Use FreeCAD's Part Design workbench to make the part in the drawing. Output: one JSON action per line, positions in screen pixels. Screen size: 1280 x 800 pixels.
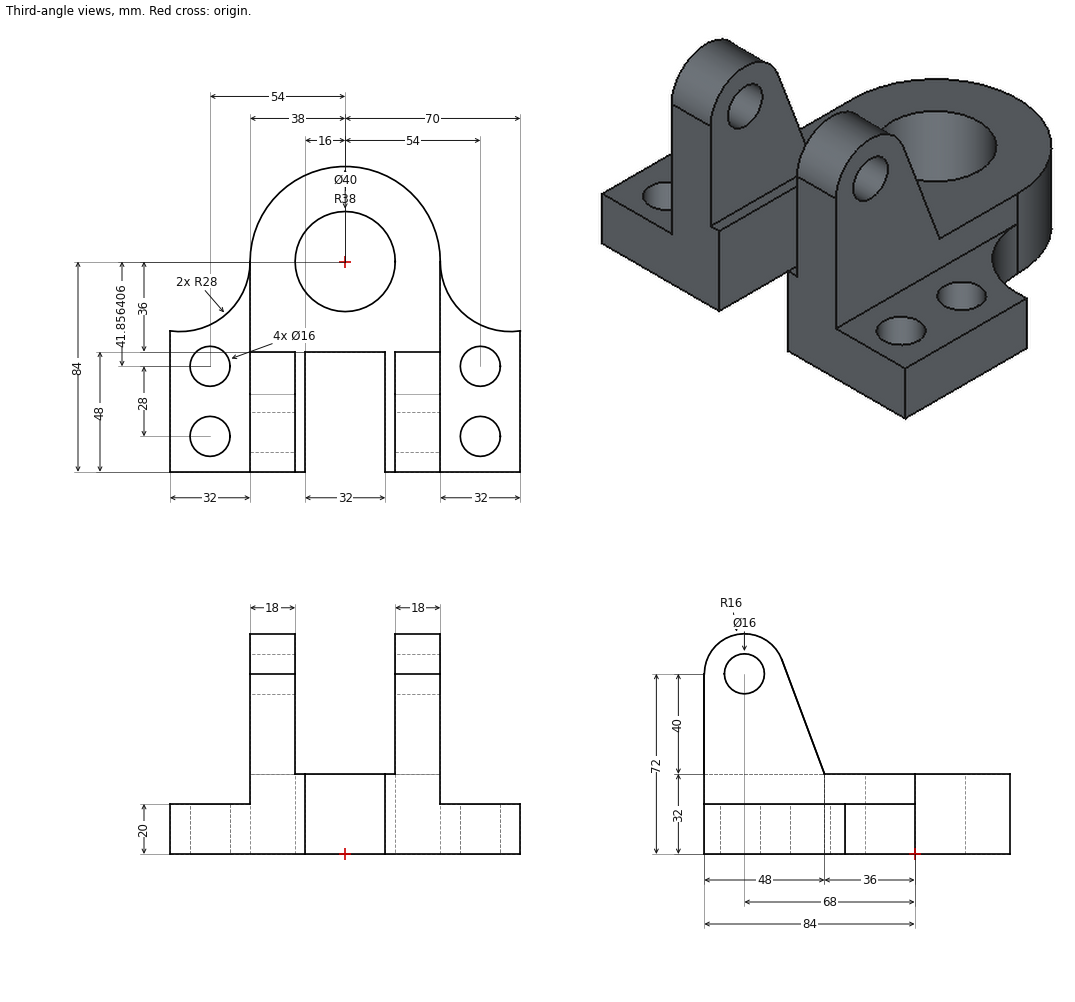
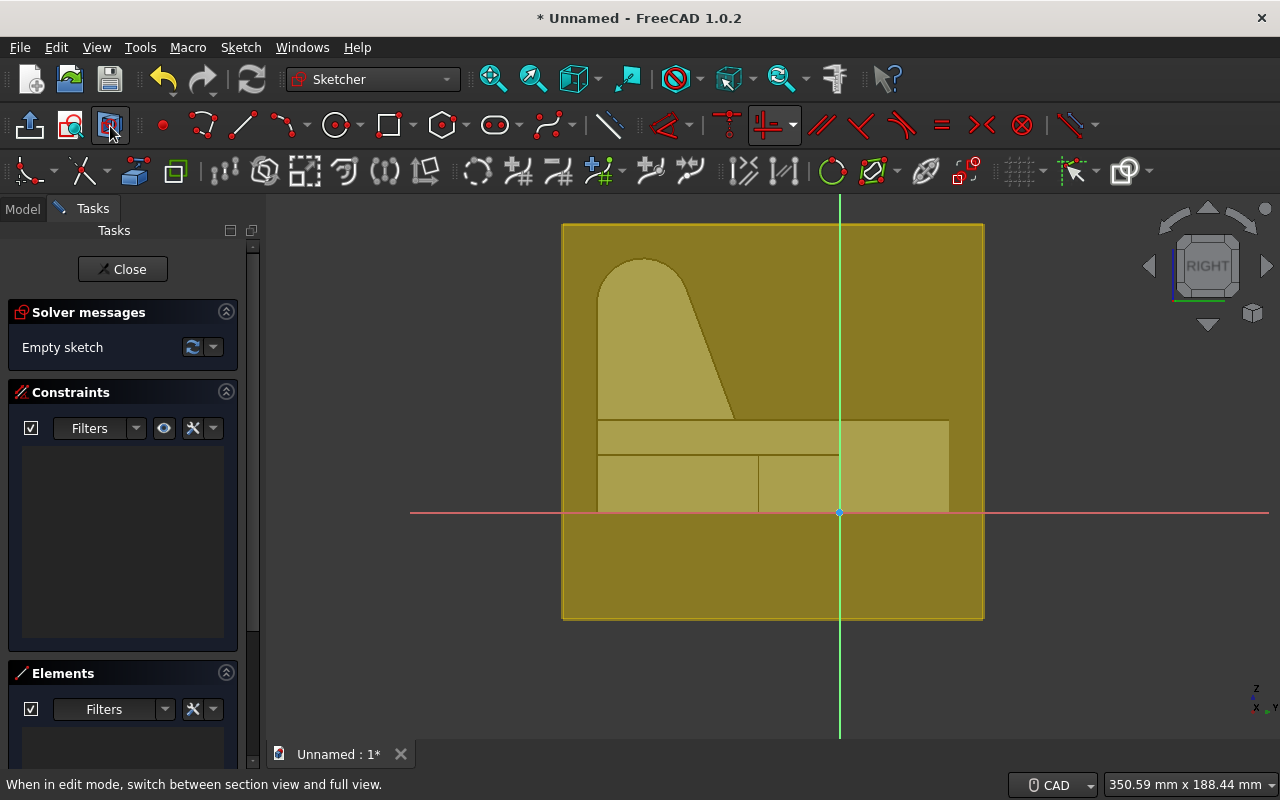
{"action": "scroll", "coordinate": [746, 222], "scroll_direction": "up", "scroll_amount": 2}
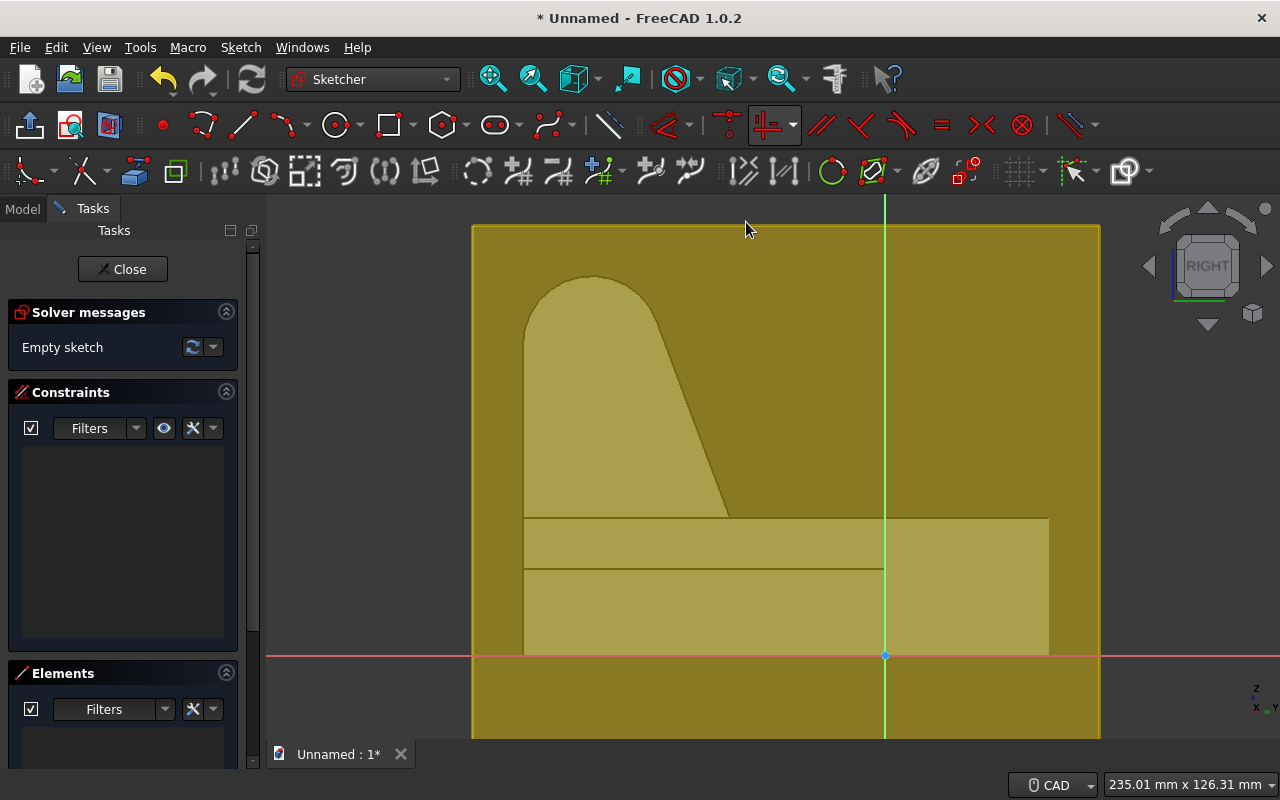
{"action": "left_click", "coordinate": [204, 126]}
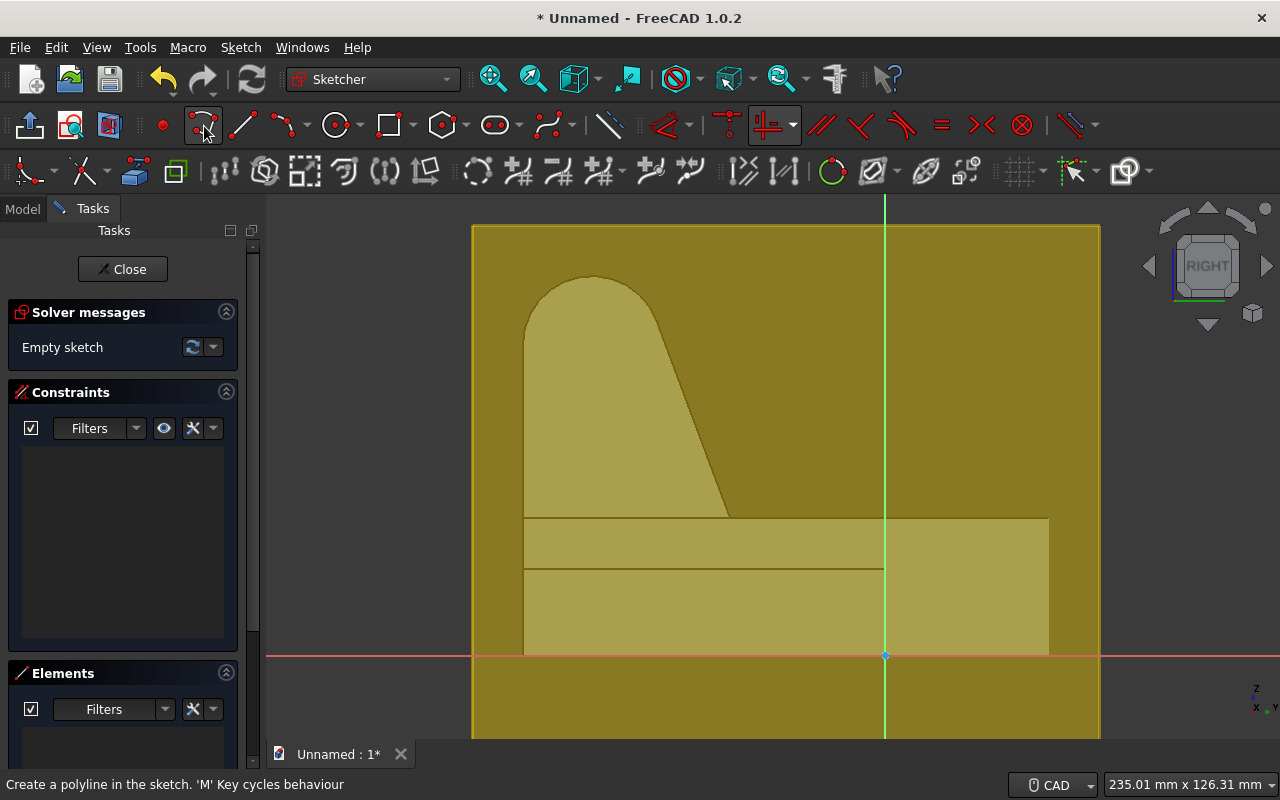
{"action": "left_click", "coordinate": [523, 345]}
{"action": "left_click", "coordinate": [523, 518]}
{"action": "left_click", "coordinate": [730, 518]}
{"action": "left_click", "coordinate": [657, 321]}
{"action": "right_click", "coordinate": [657, 321]}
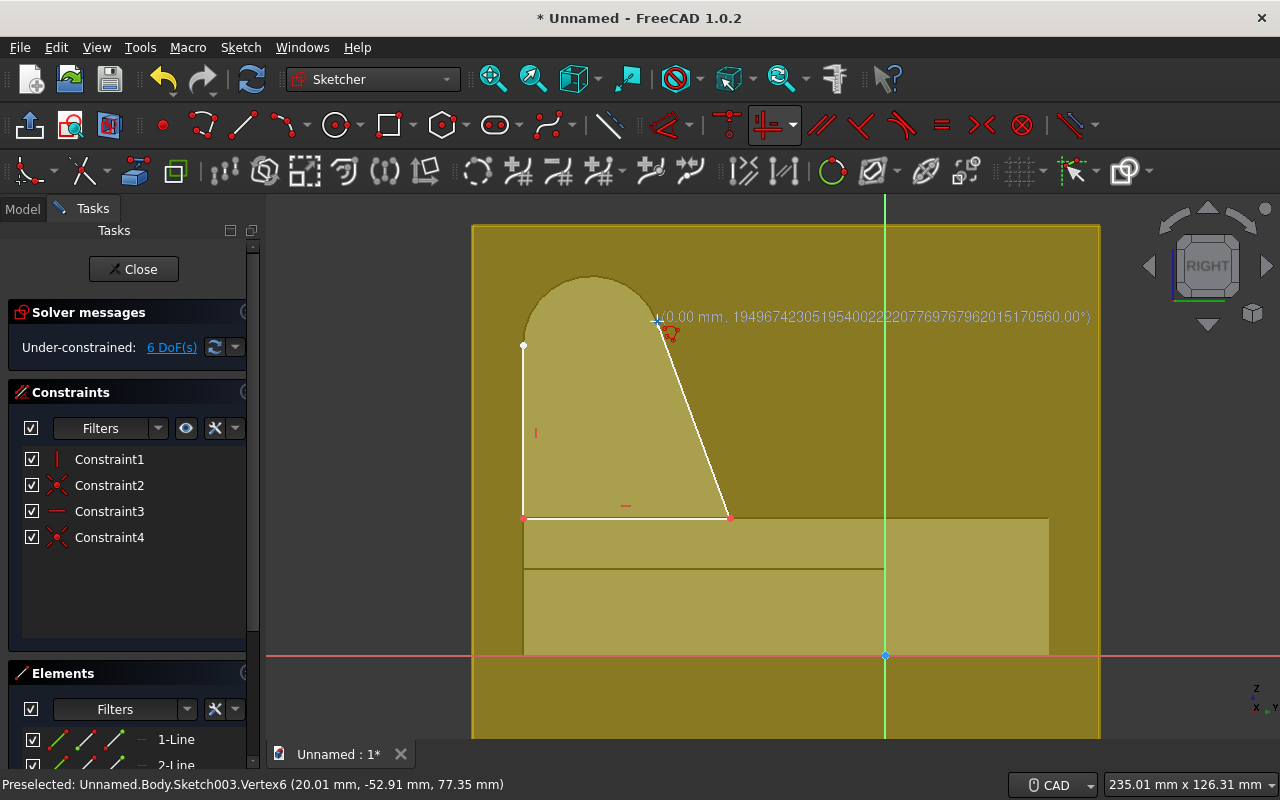
{"action": "left_click", "coordinate": [284, 126]}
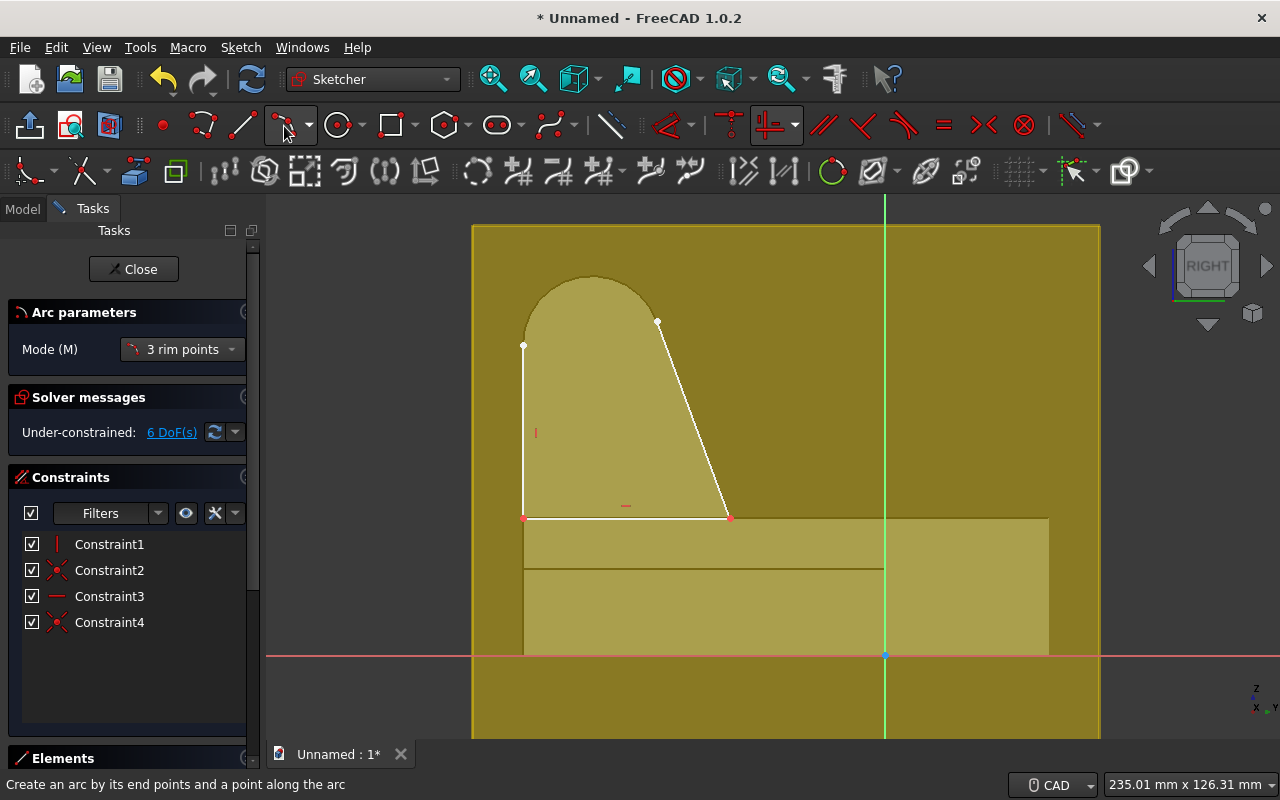
{"action": "left_click", "coordinate": [657, 322]}
{"action": "left_click", "coordinate": [523, 346]}
{"action": "left_click", "coordinate": [580, 277]}
{"action": "key", "text": "Escape"}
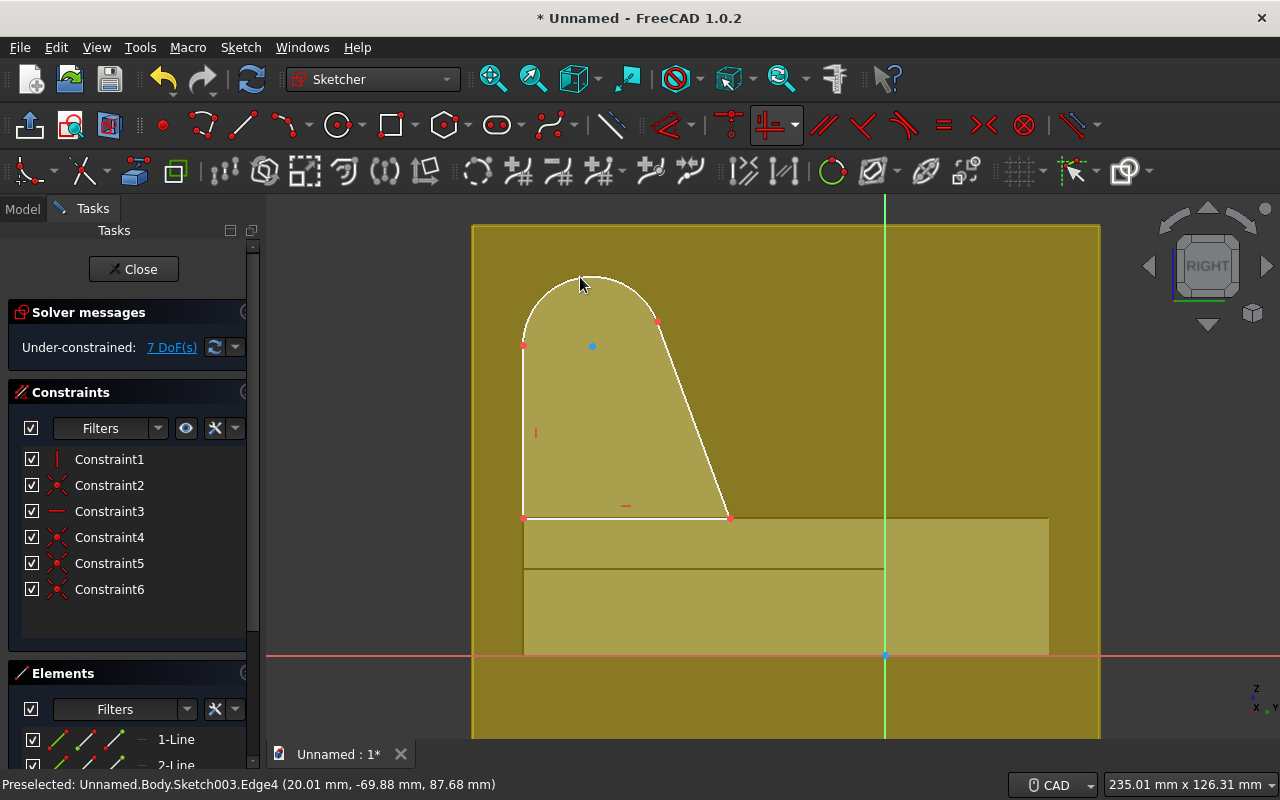
{"action": "left_click", "coordinate": [523, 398]}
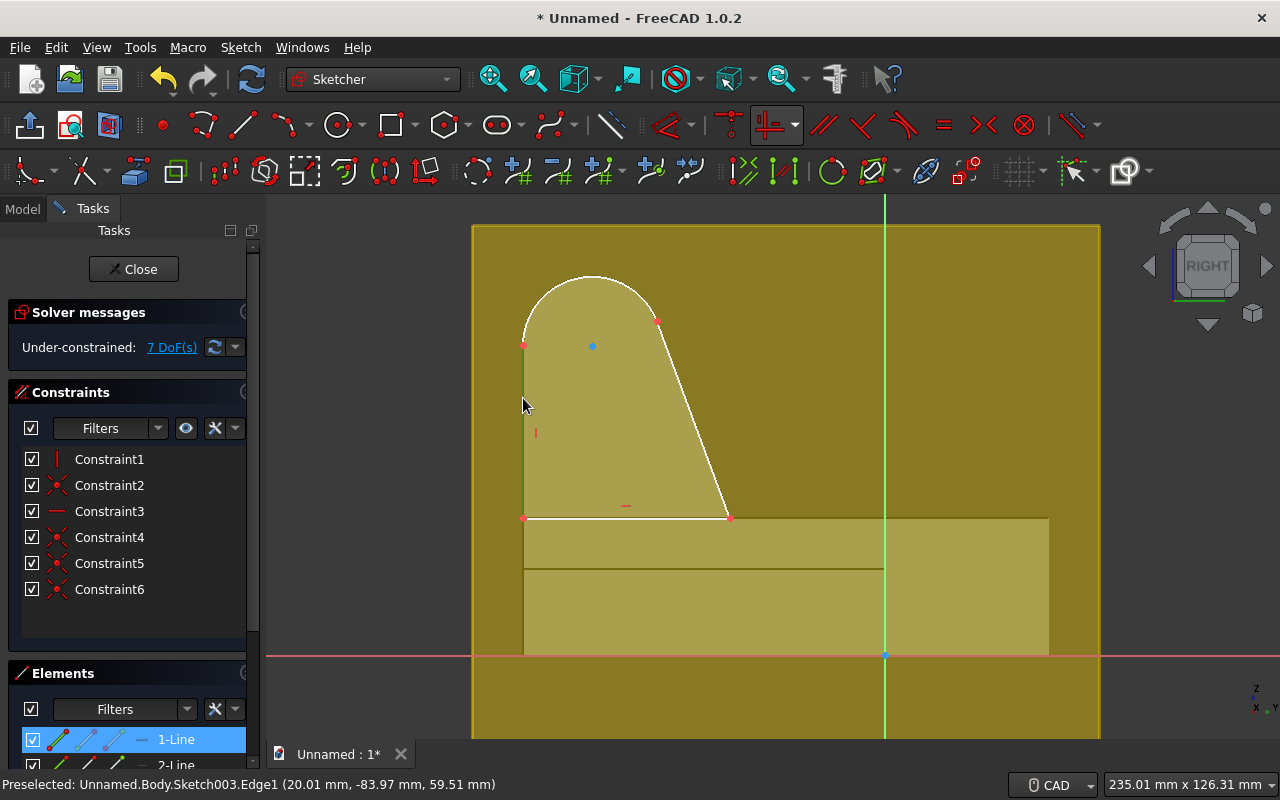
{"action": "left_click", "coordinate": [618, 282]}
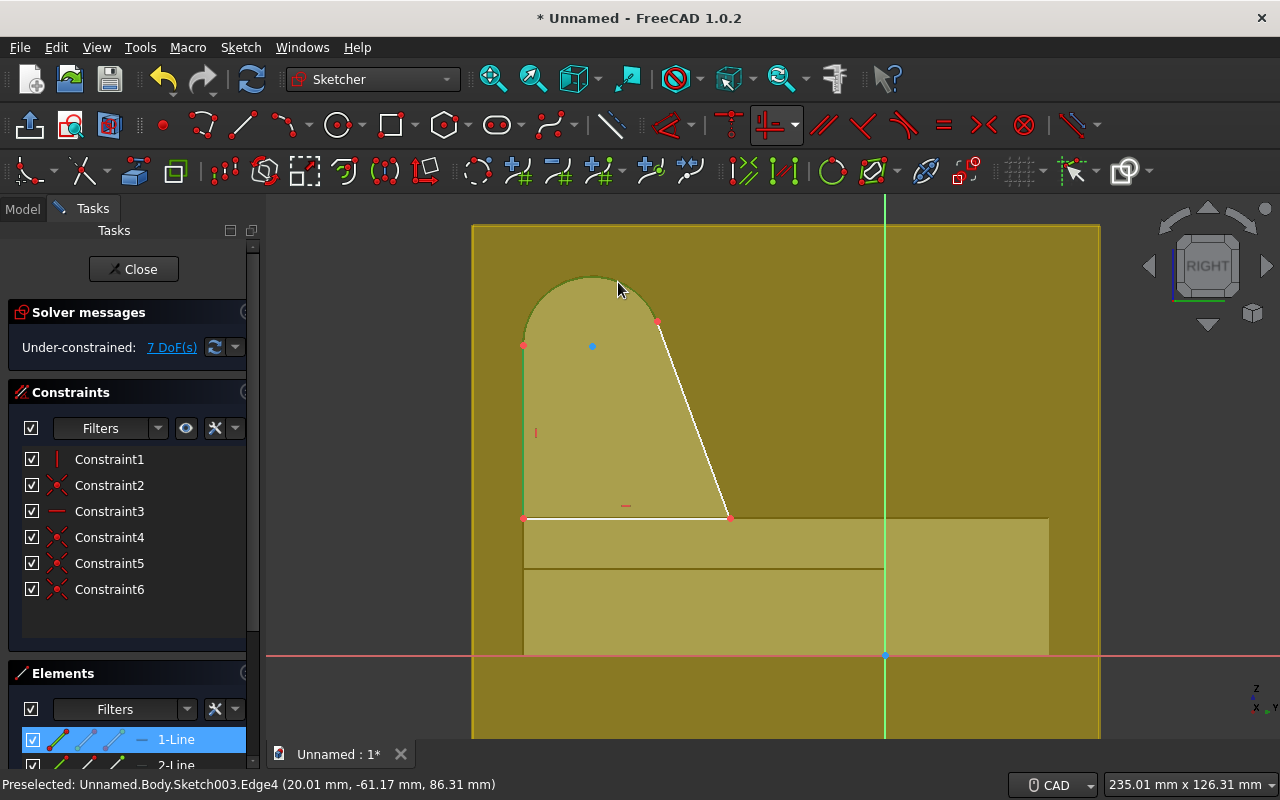
{"action": "left_click", "coordinate": [904, 126]}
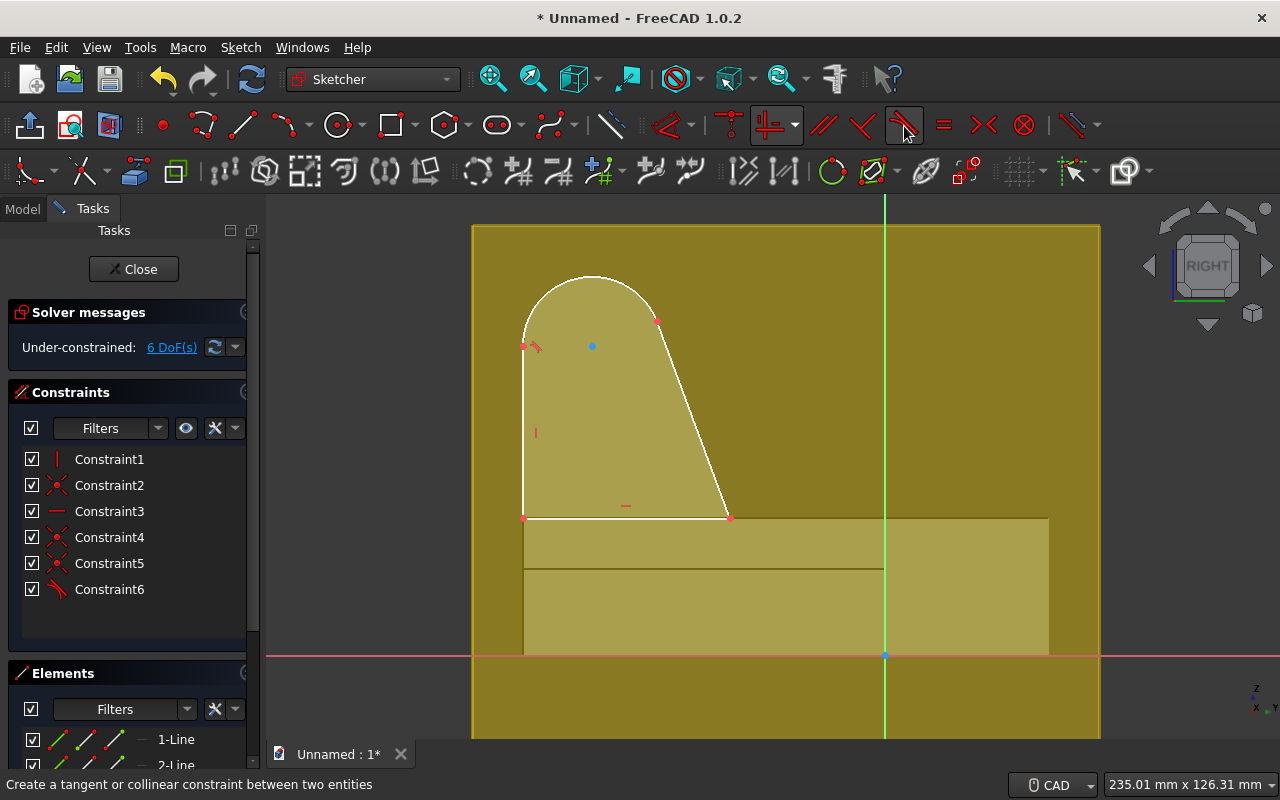
{"action": "left_click", "coordinate": [708, 460]}